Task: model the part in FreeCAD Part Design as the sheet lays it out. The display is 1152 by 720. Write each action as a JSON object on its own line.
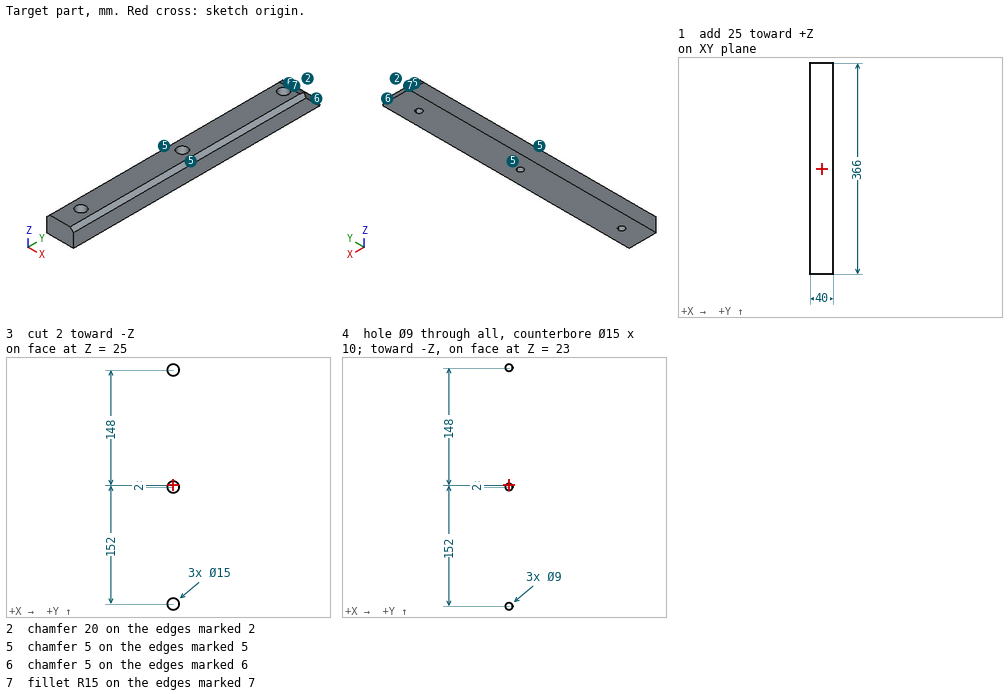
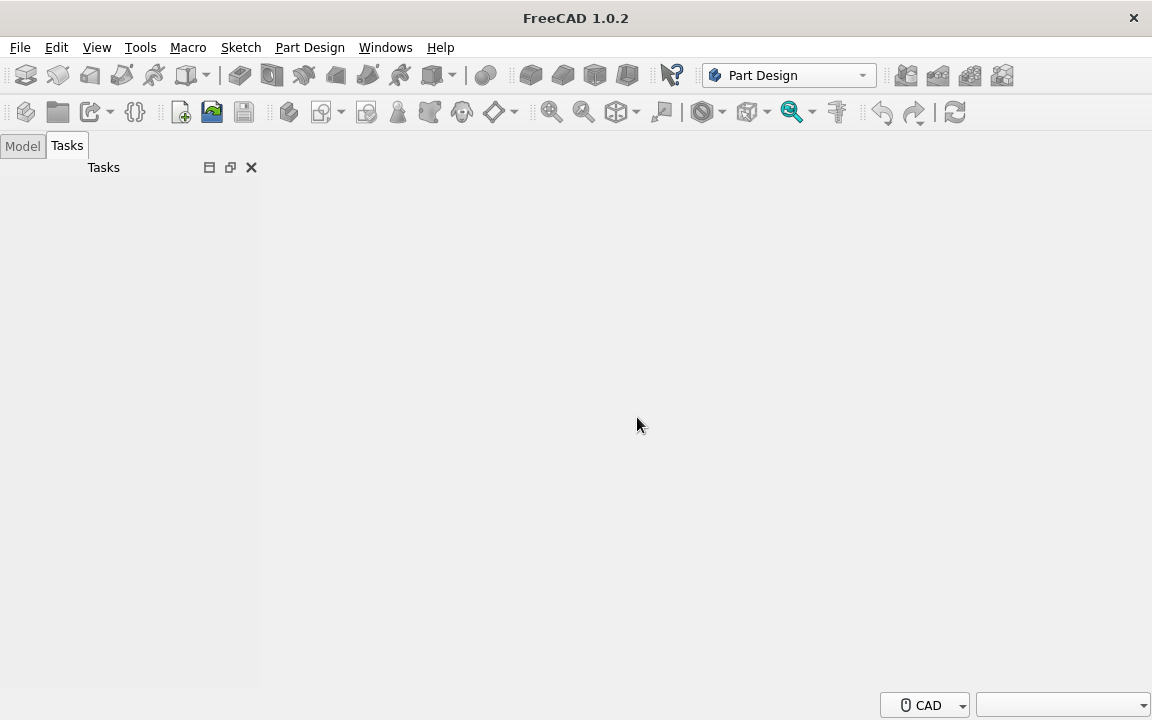
{"action": "left_click", "coordinate": [180, 112]}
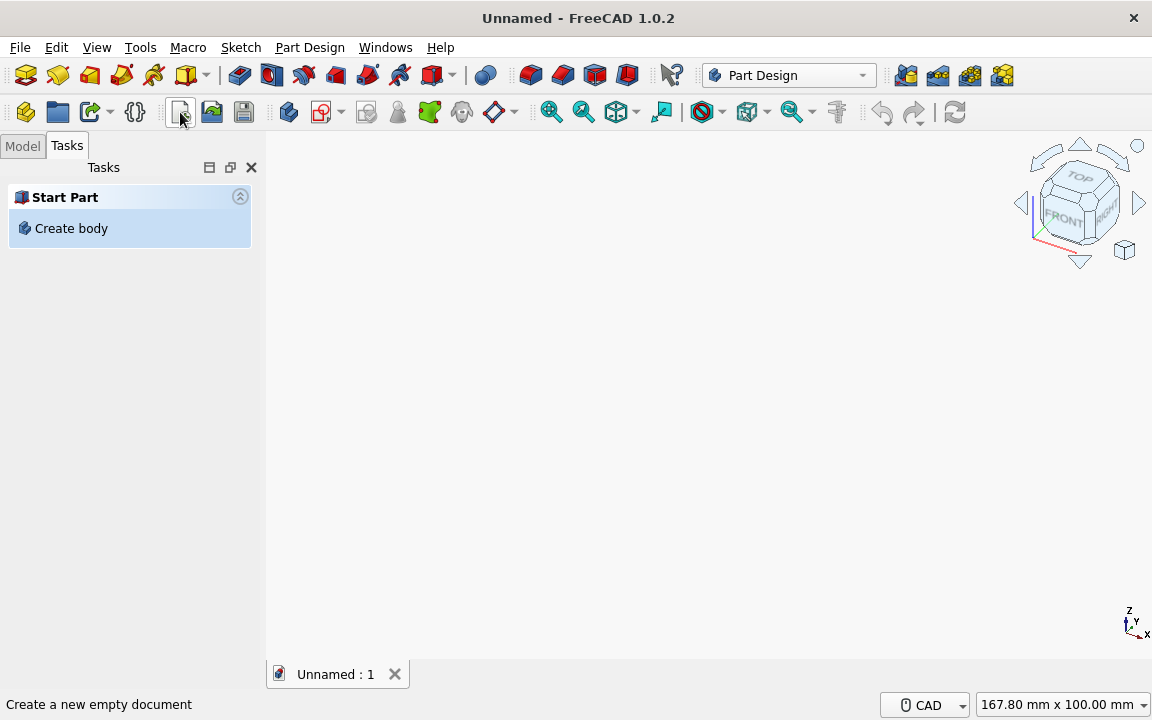
{"action": "left_click", "coordinate": [322, 112]}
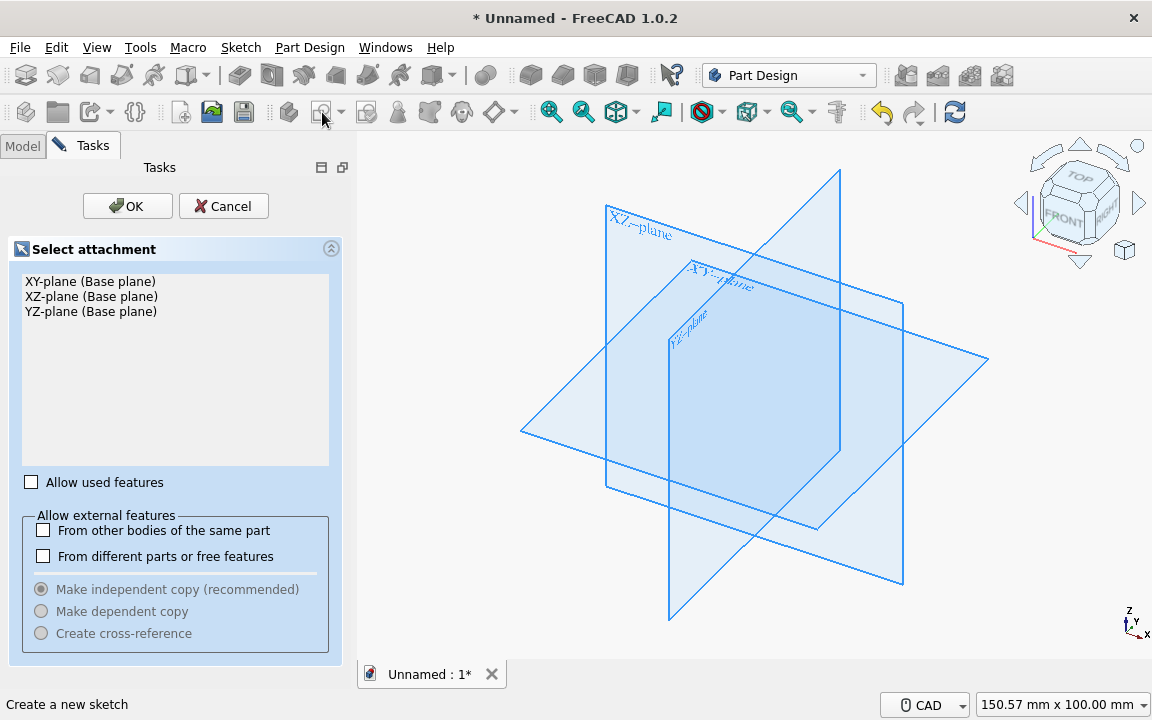
{"action": "left_click", "coordinate": [82, 282]}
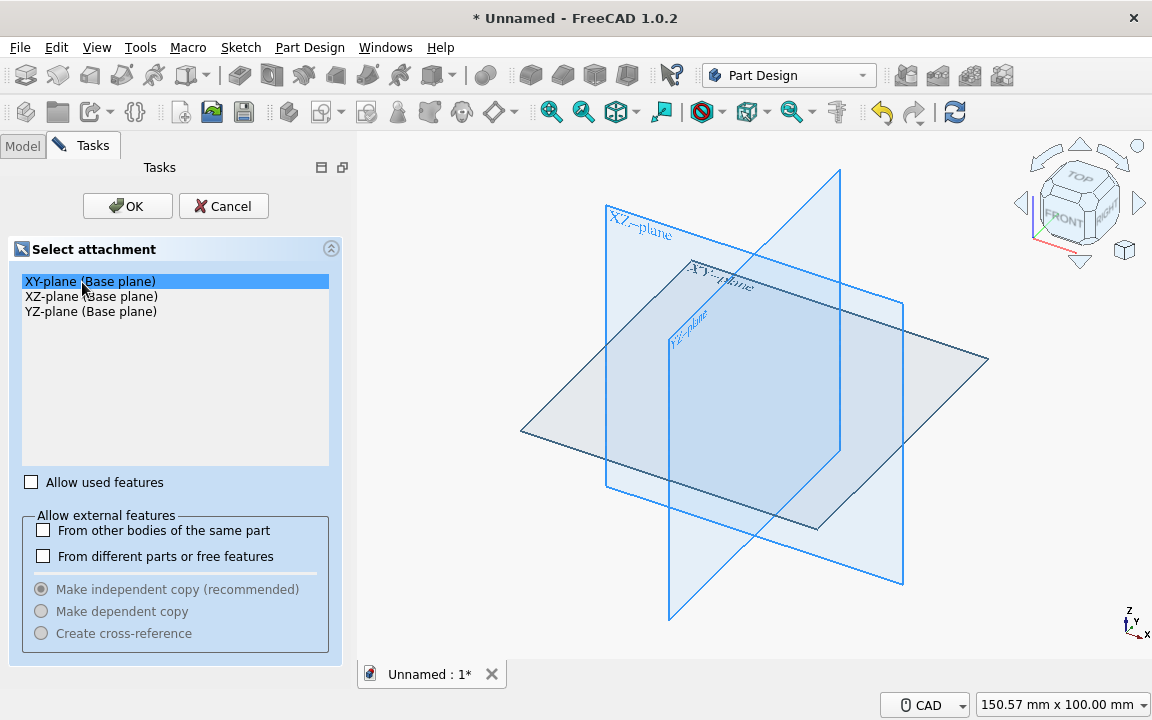
{"action": "left_click", "coordinate": [128, 206]}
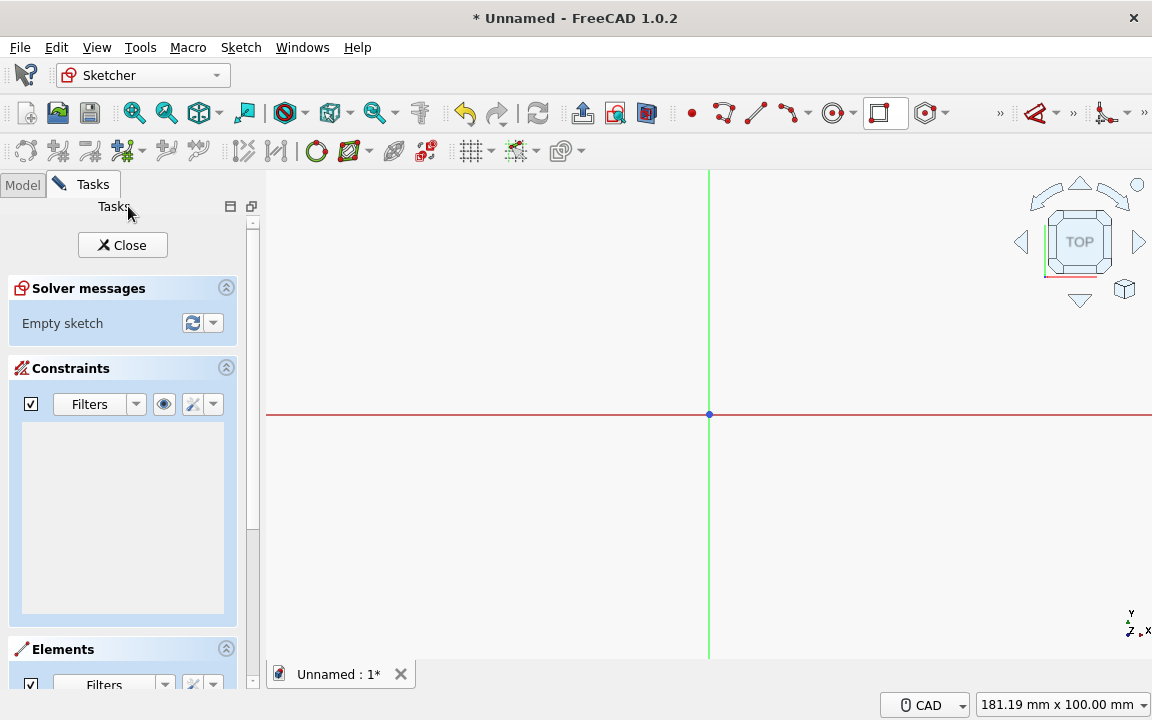
{"action": "scroll", "coordinate": [627, 415], "scroll_direction": "down", "scroll_amount": 9}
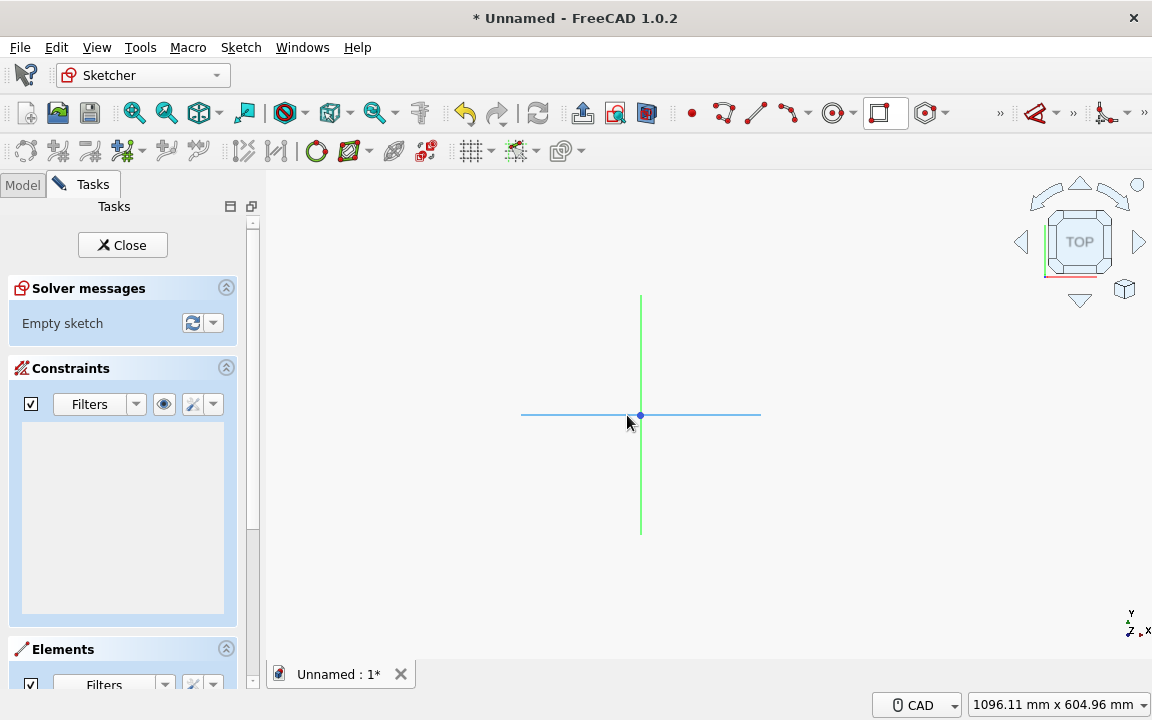
{"action": "left_click", "coordinate": [902, 114]}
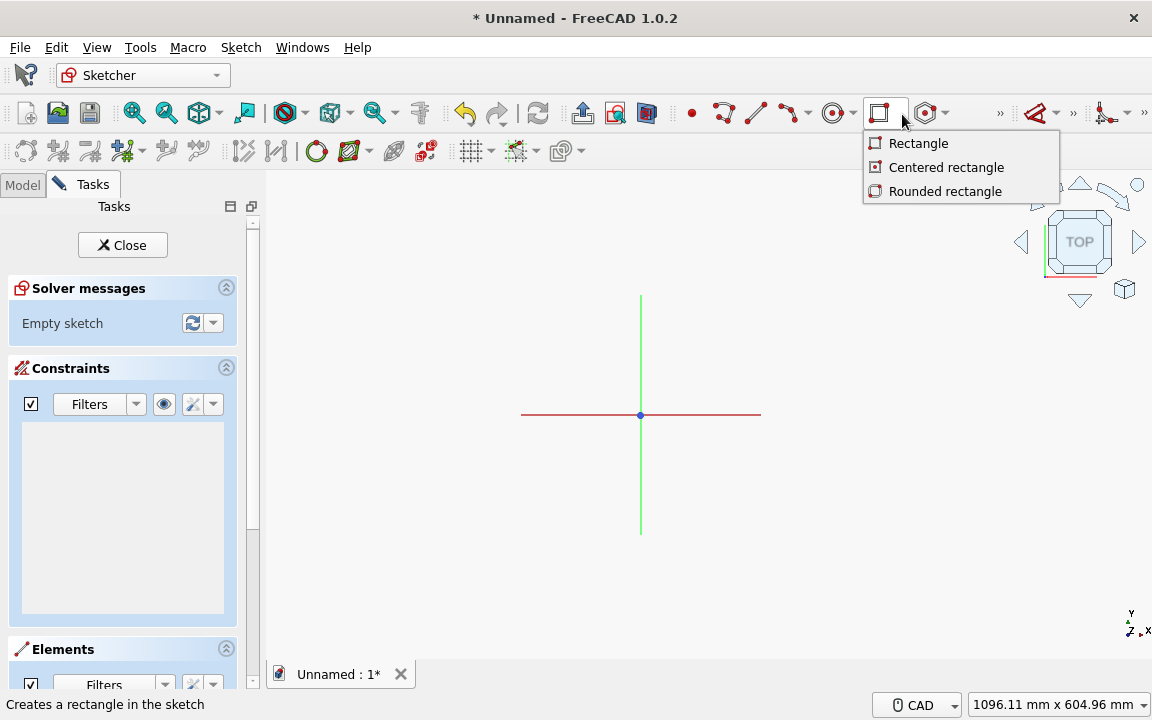
{"action": "left_click", "coordinate": [962, 167]}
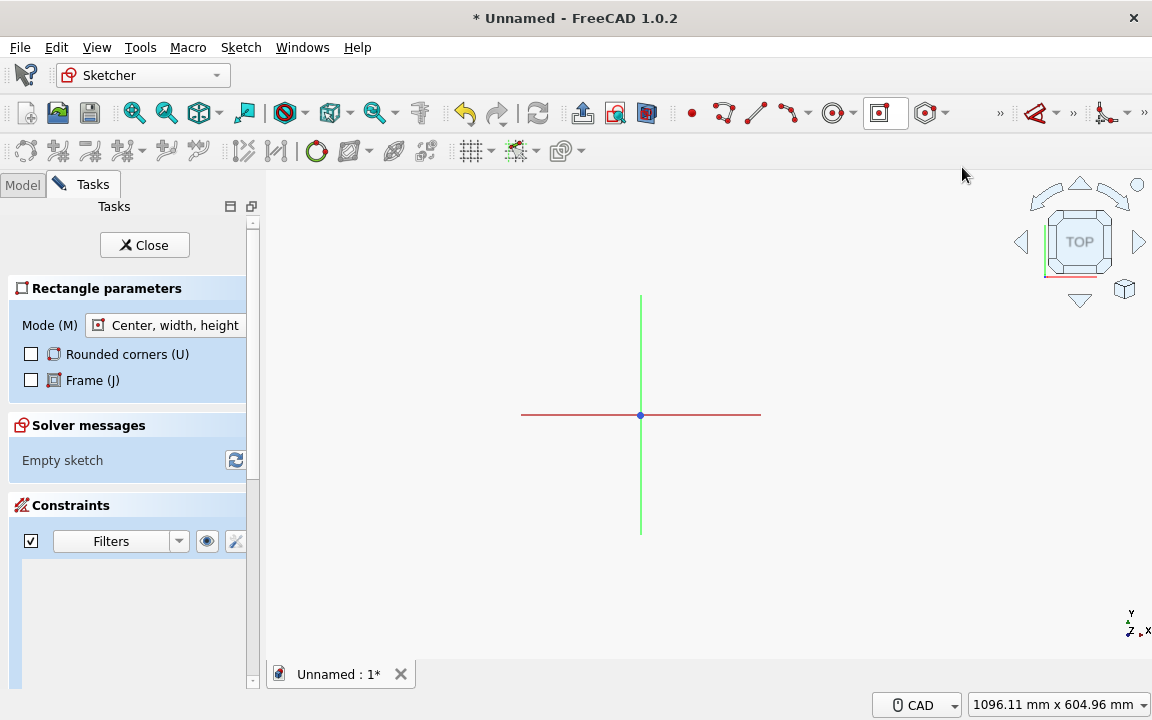
{"action": "left_click", "coordinate": [641, 415]}
{"action": "left_click", "coordinate": [657, 267]}
{"action": "key", "text": "Escape"}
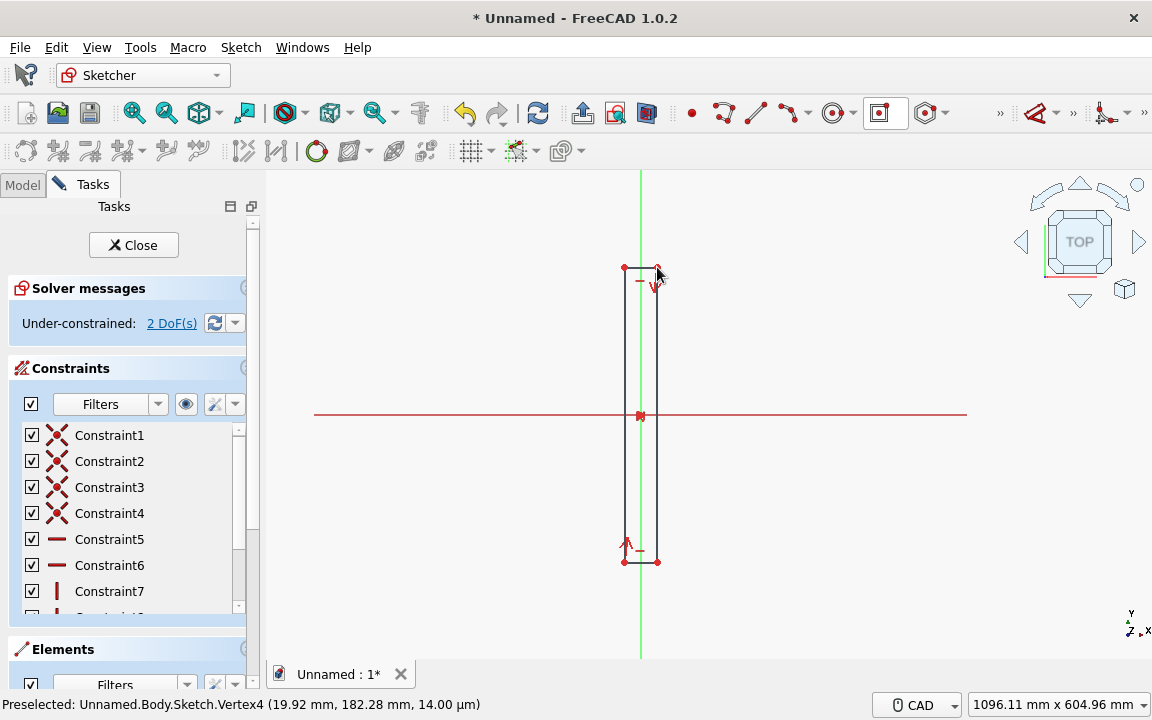
{"action": "key", "text": "d"}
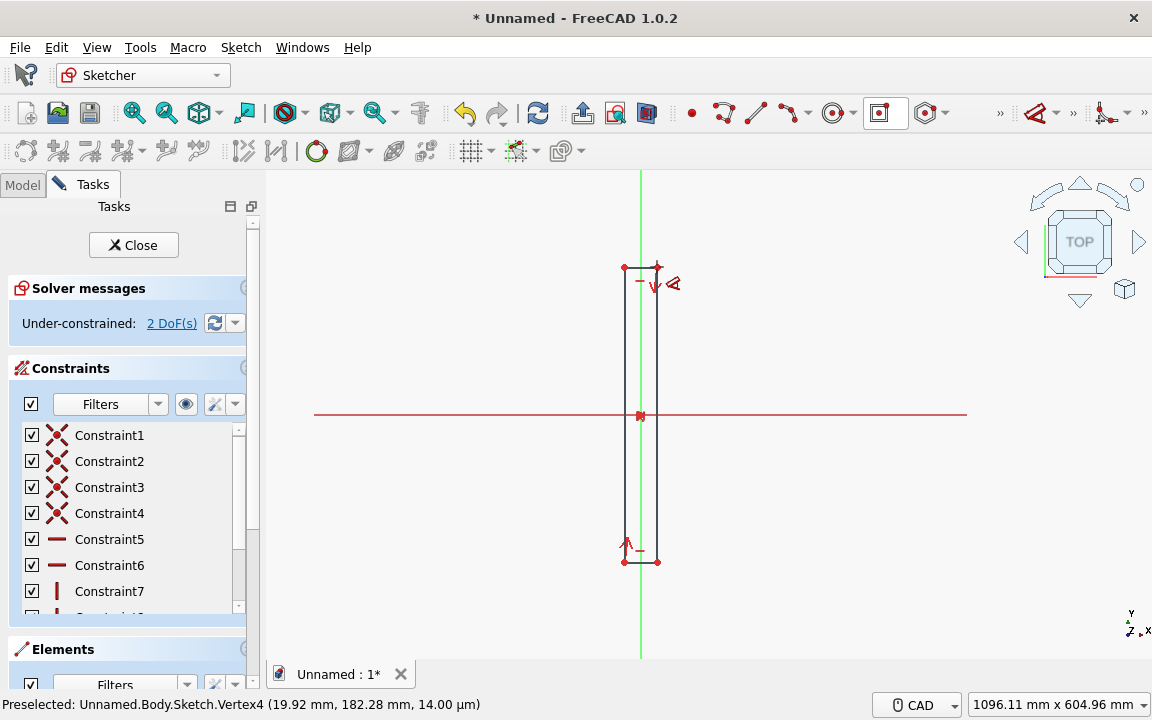
{"action": "scroll", "coordinate": [638, 563], "scroll_direction": "up", "scroll_amount": 2}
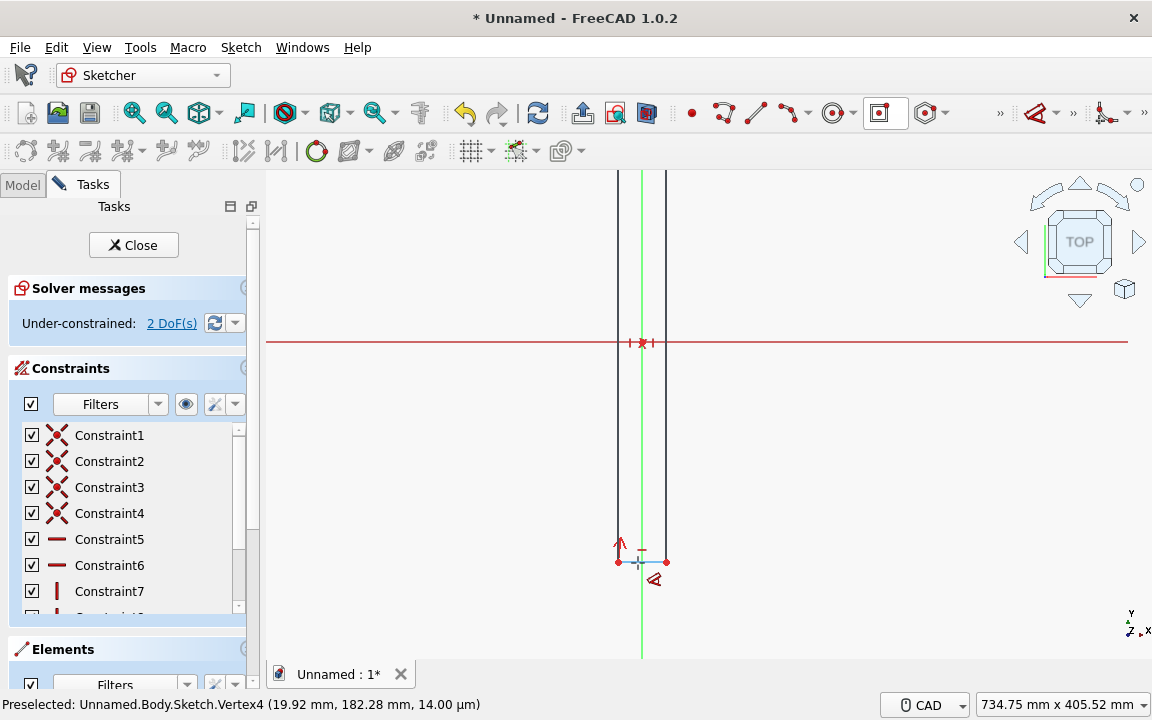
{"action": "left_click", "coordinate": [637, 562]}
{"action": "left_click", "coordinate": [625, 596]}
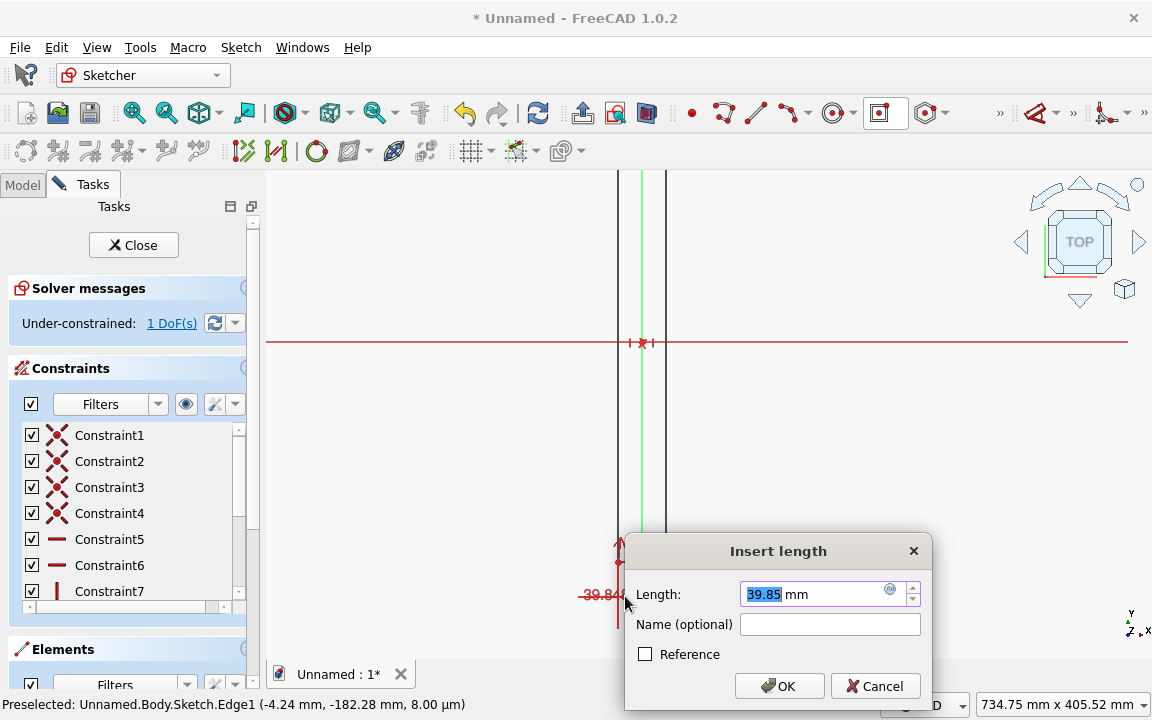
{"action": "type", "text": "40"}
{"action": "key", "text": "Return"}